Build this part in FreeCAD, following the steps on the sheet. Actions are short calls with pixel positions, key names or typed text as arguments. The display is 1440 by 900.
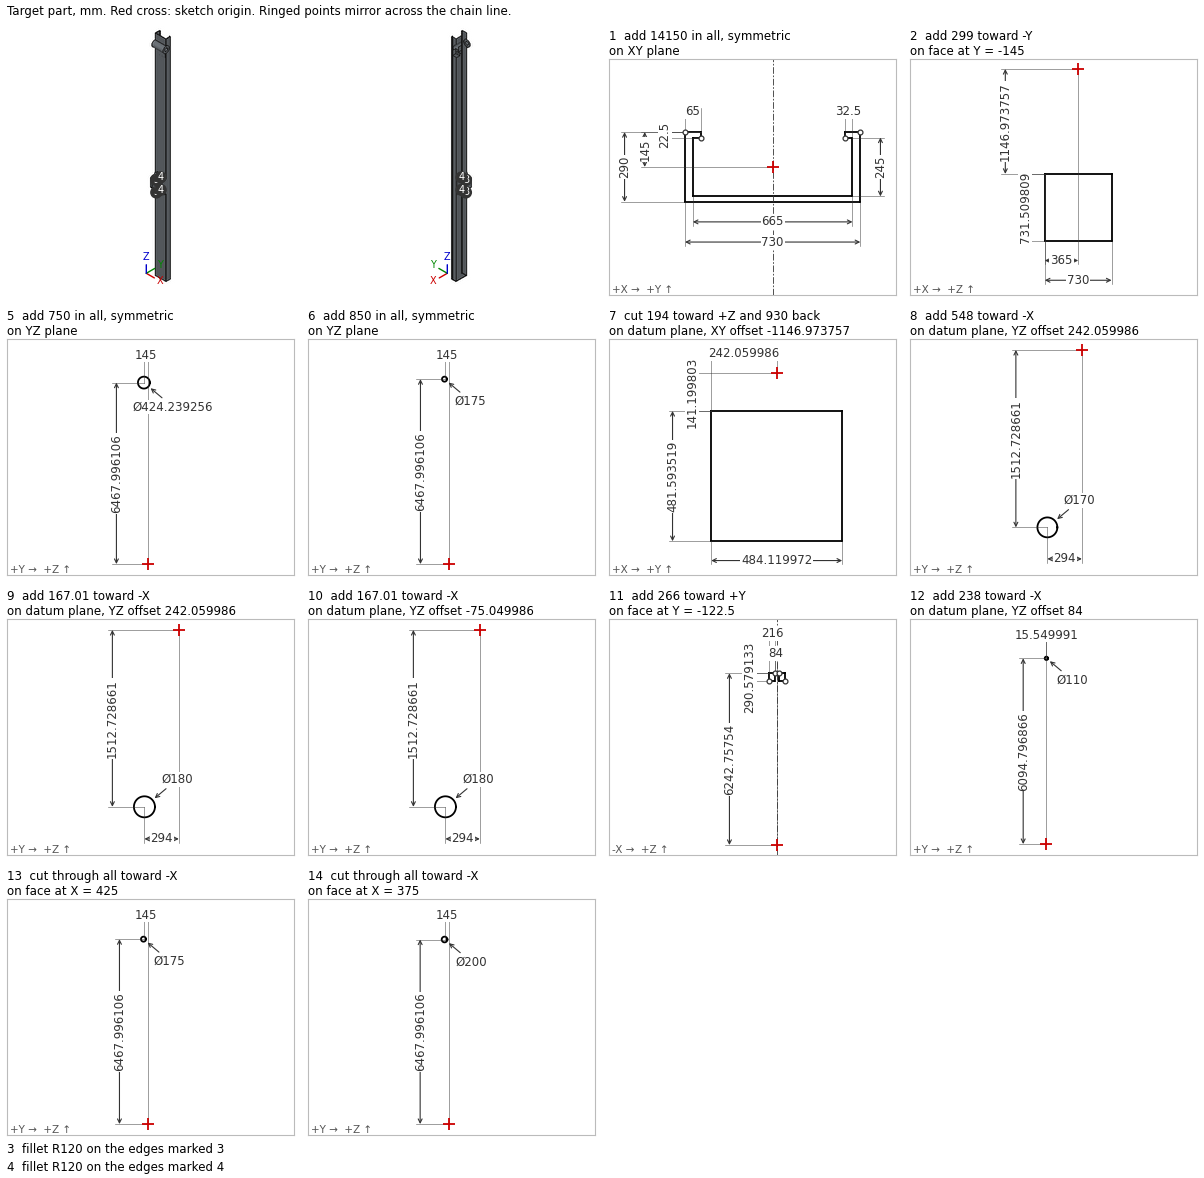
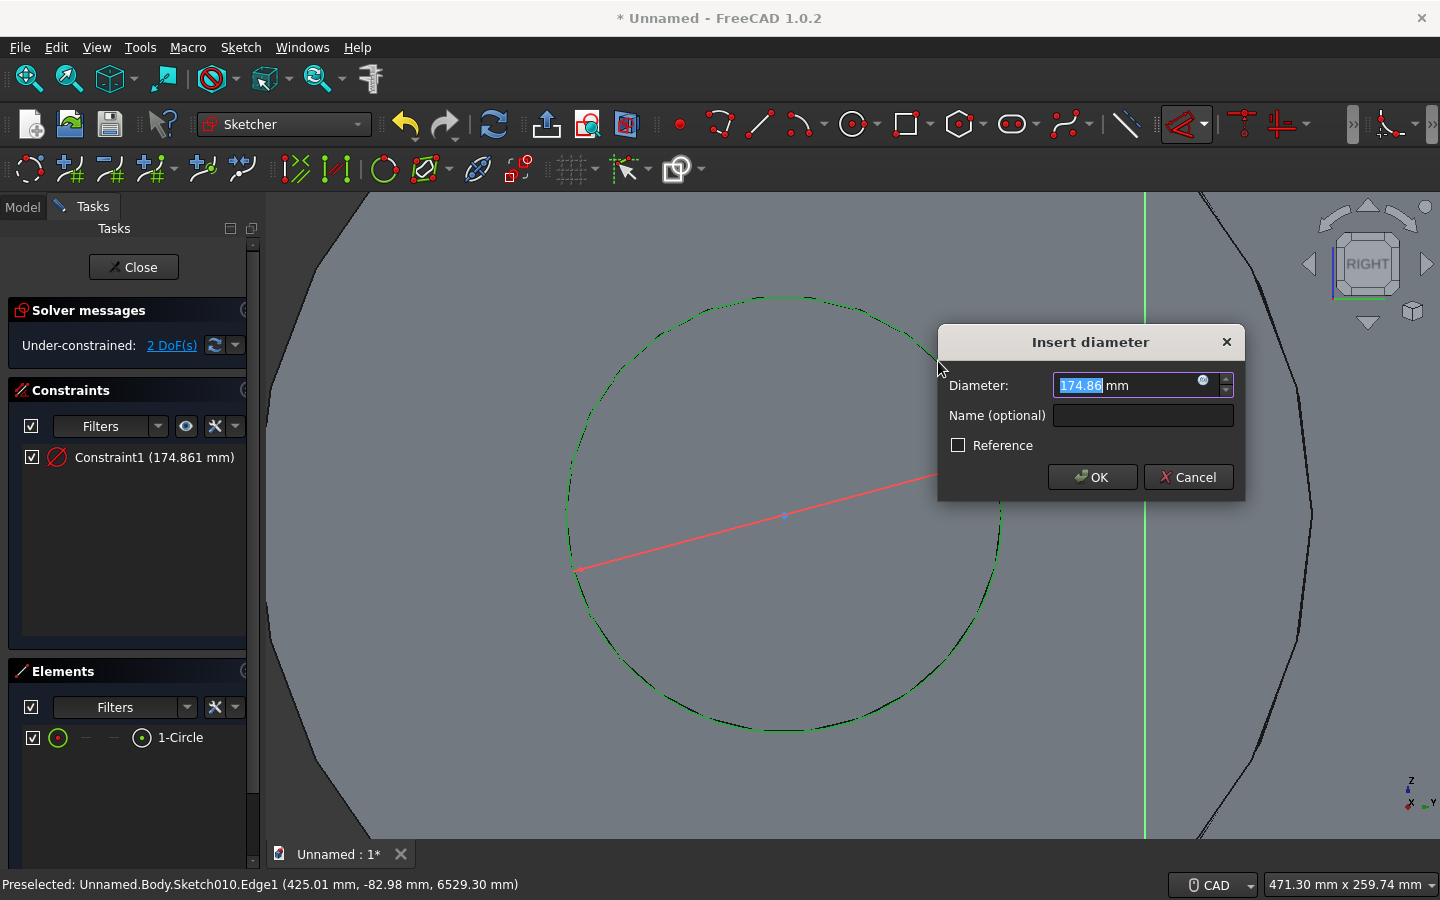
text(175)
key(Return)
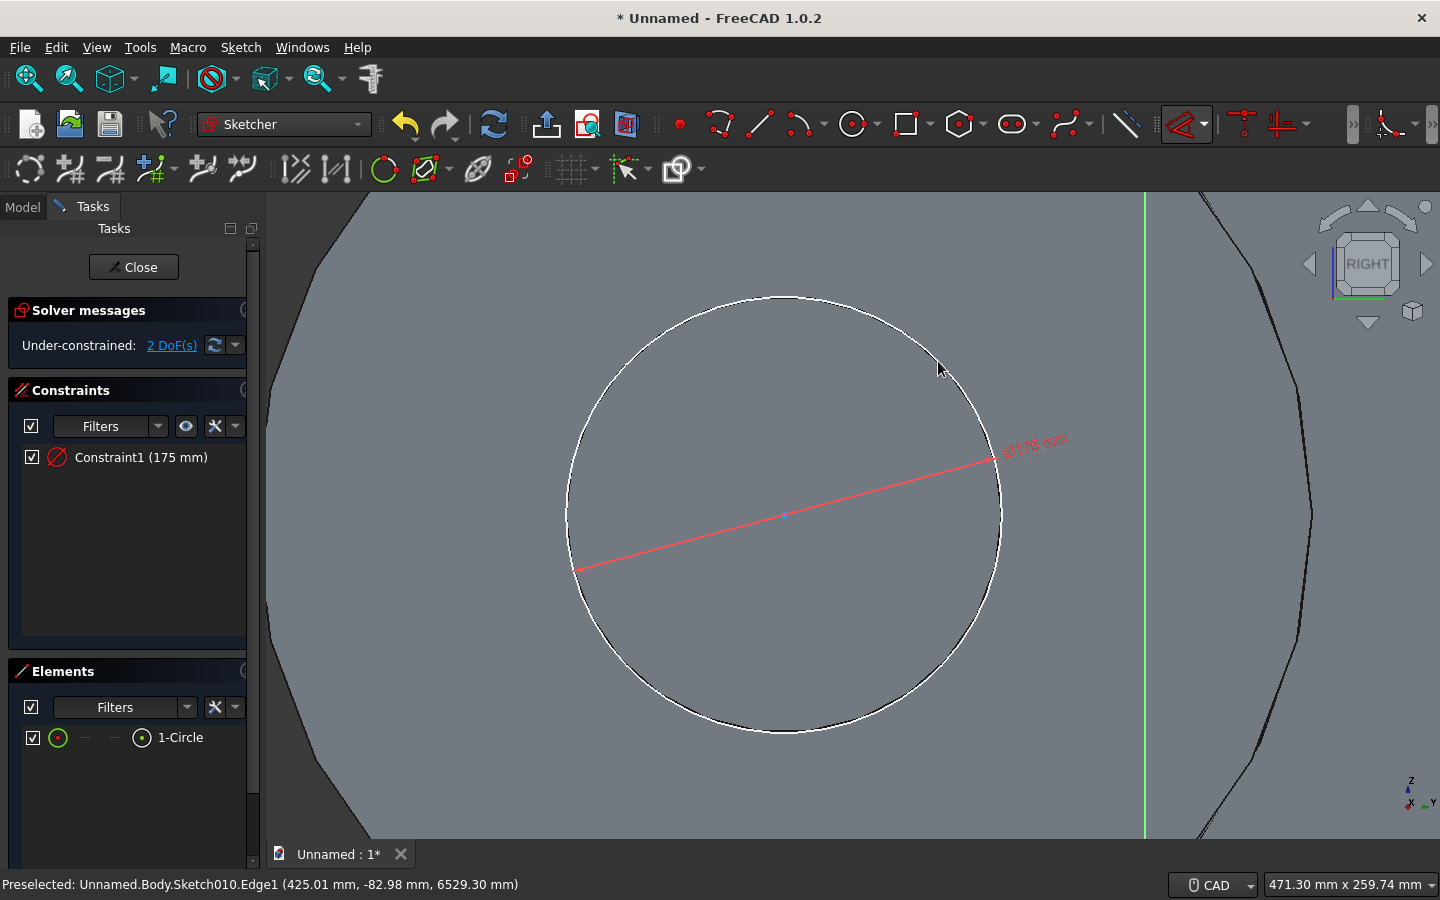
click(784, 515)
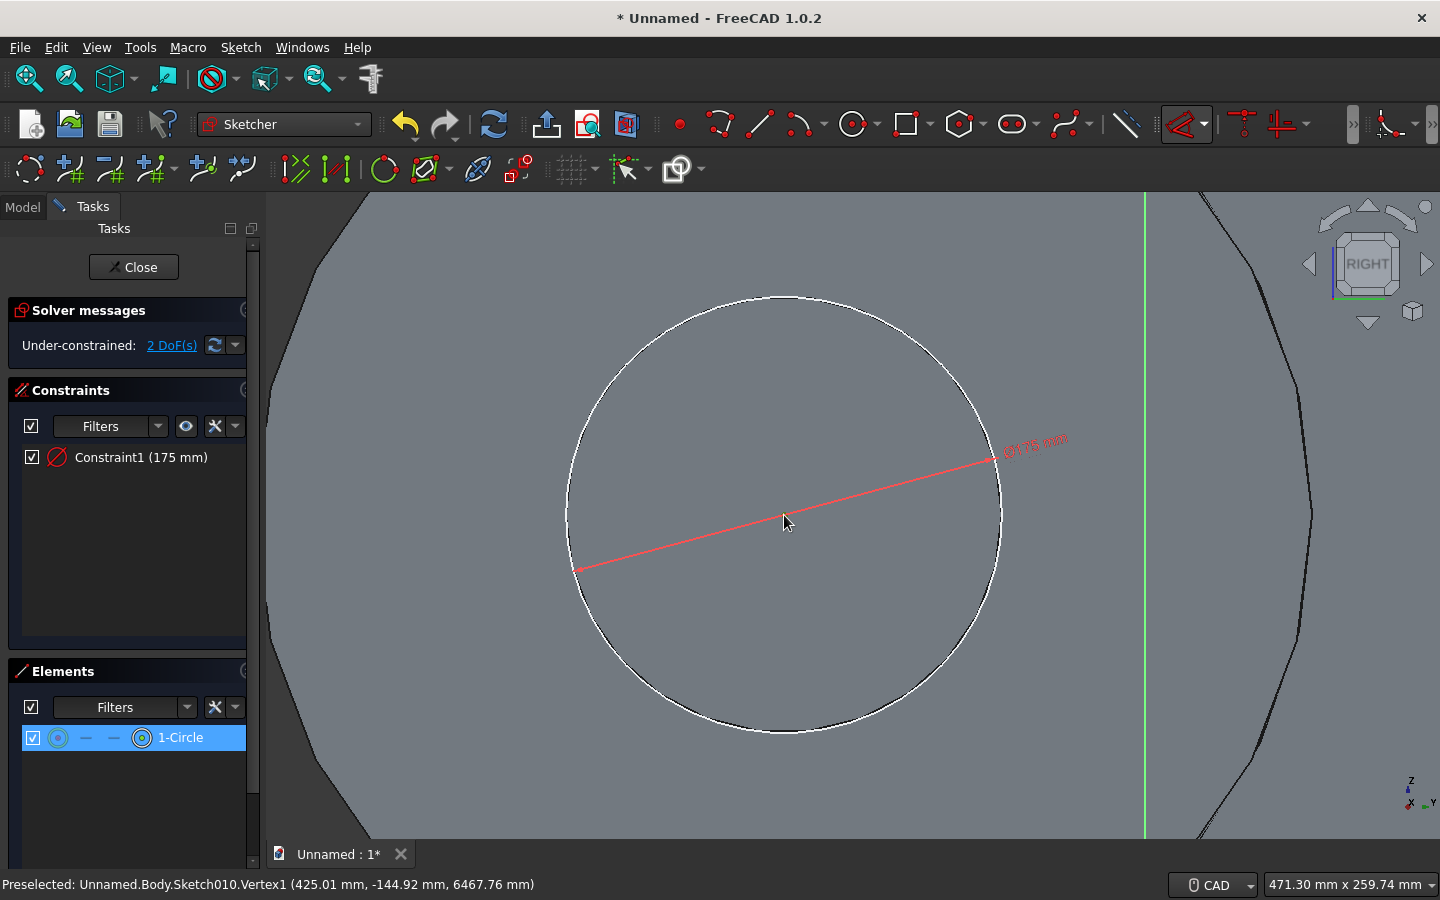
key(l)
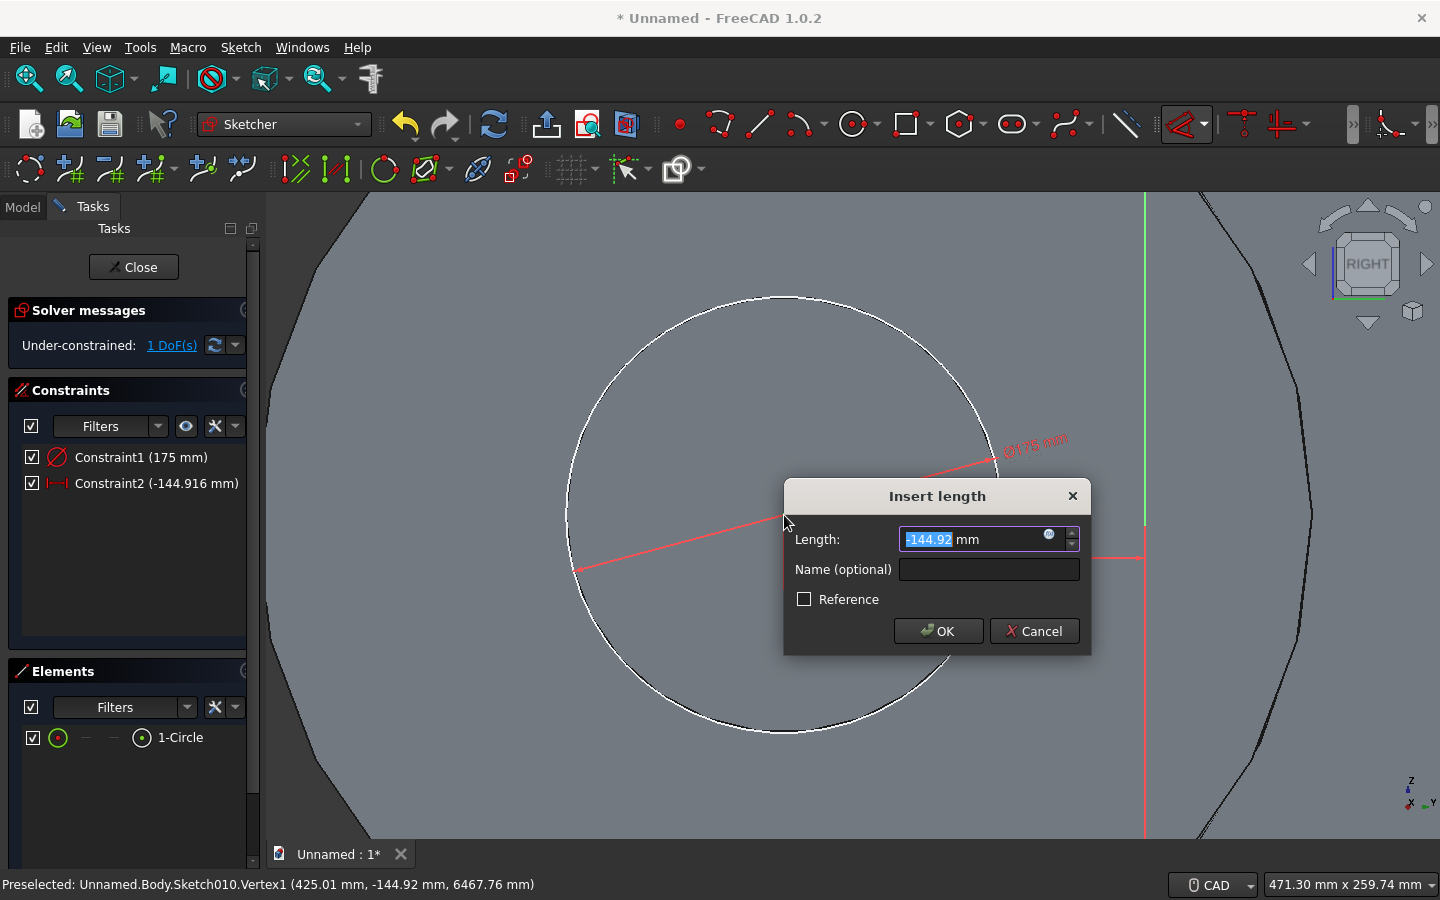
text(-145)
key(Return)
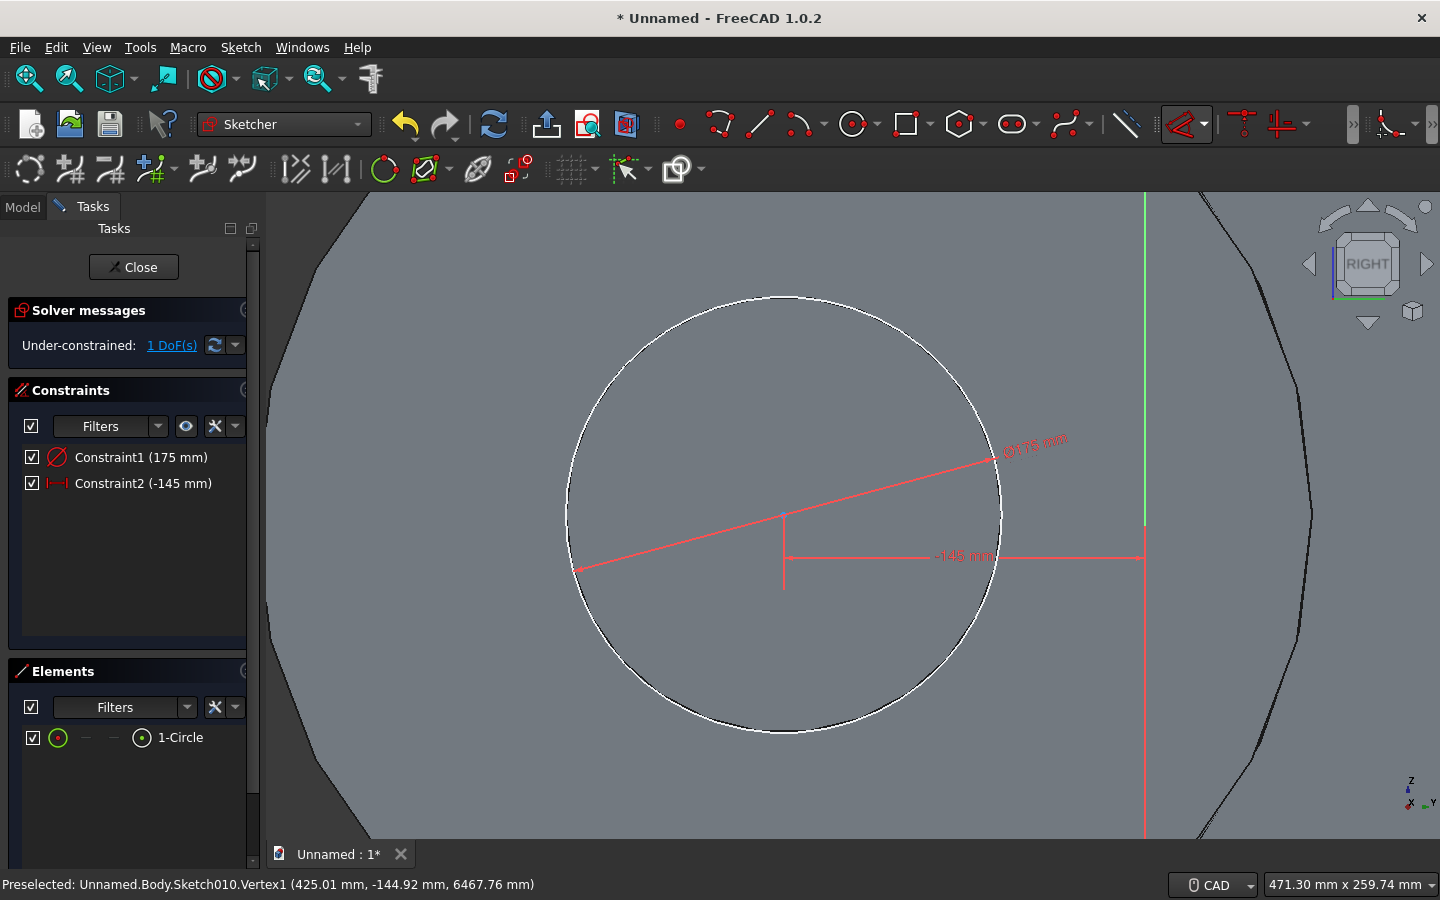
click(782, 517)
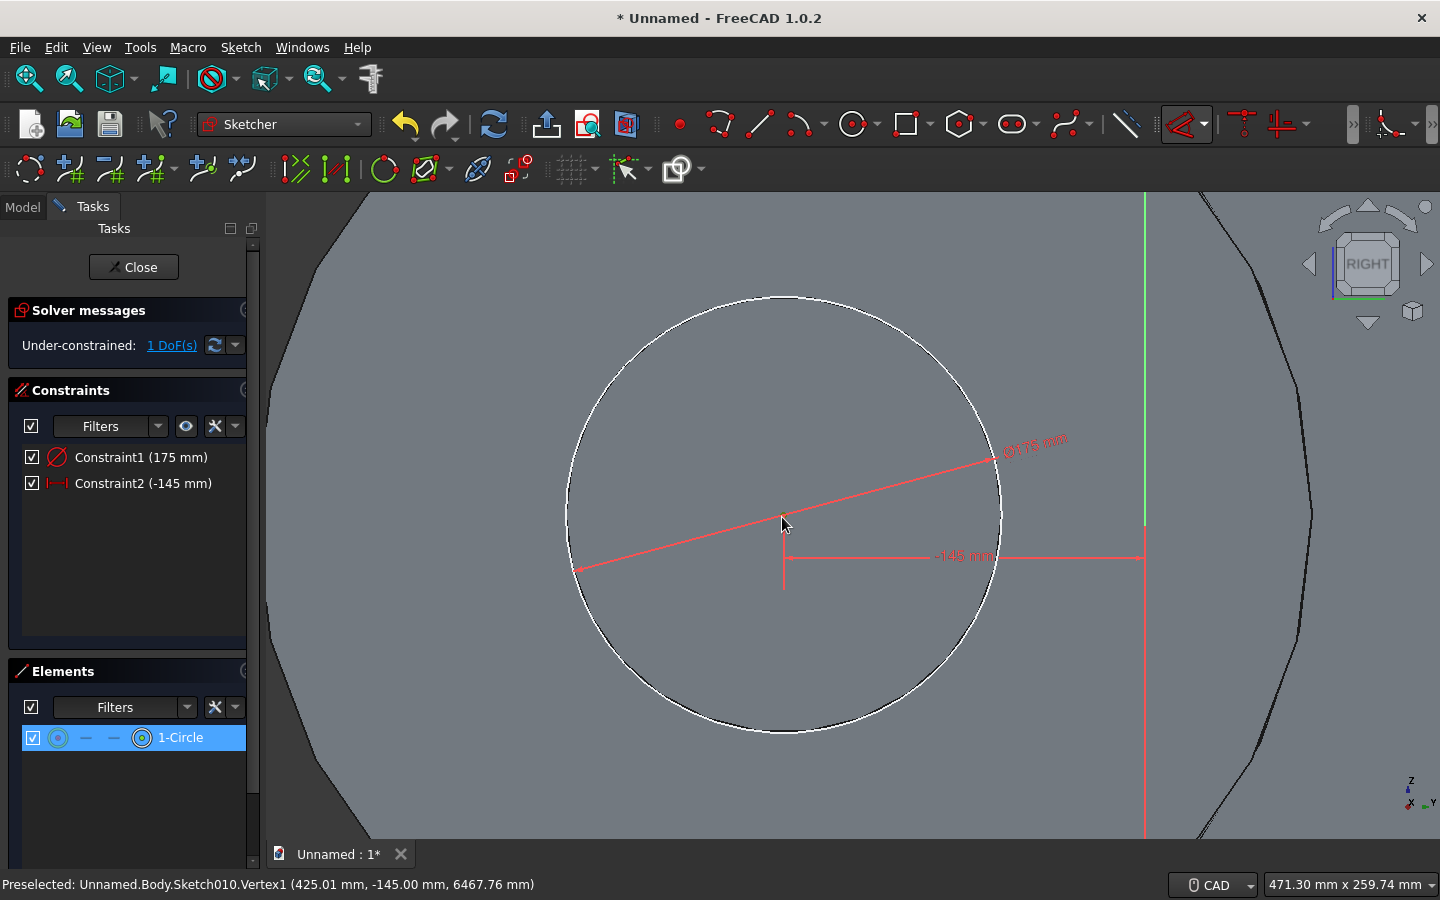
key(i)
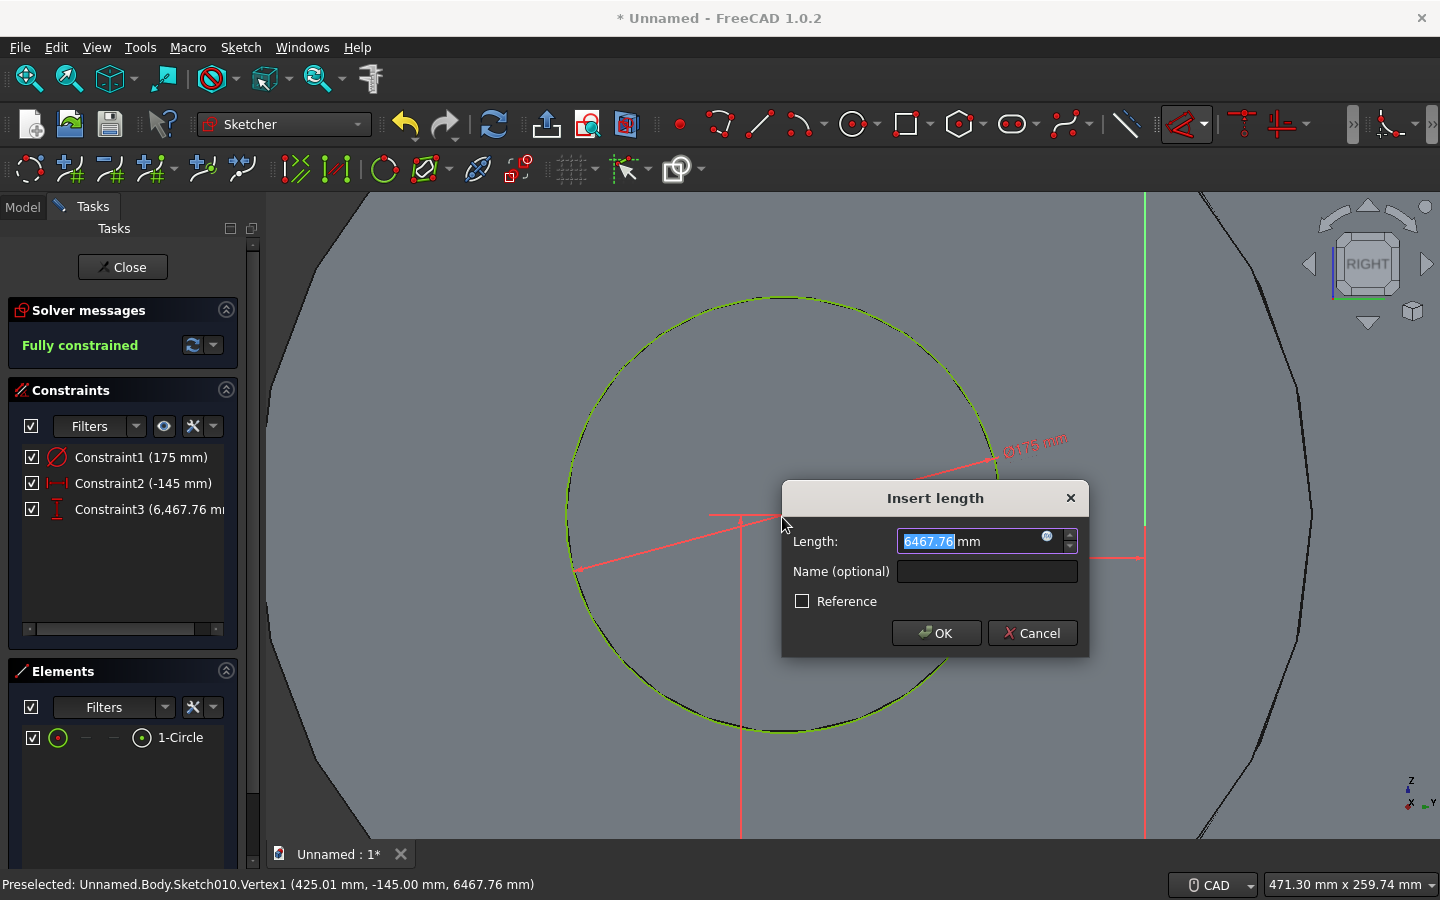
text(6467.996106)
key(Return)